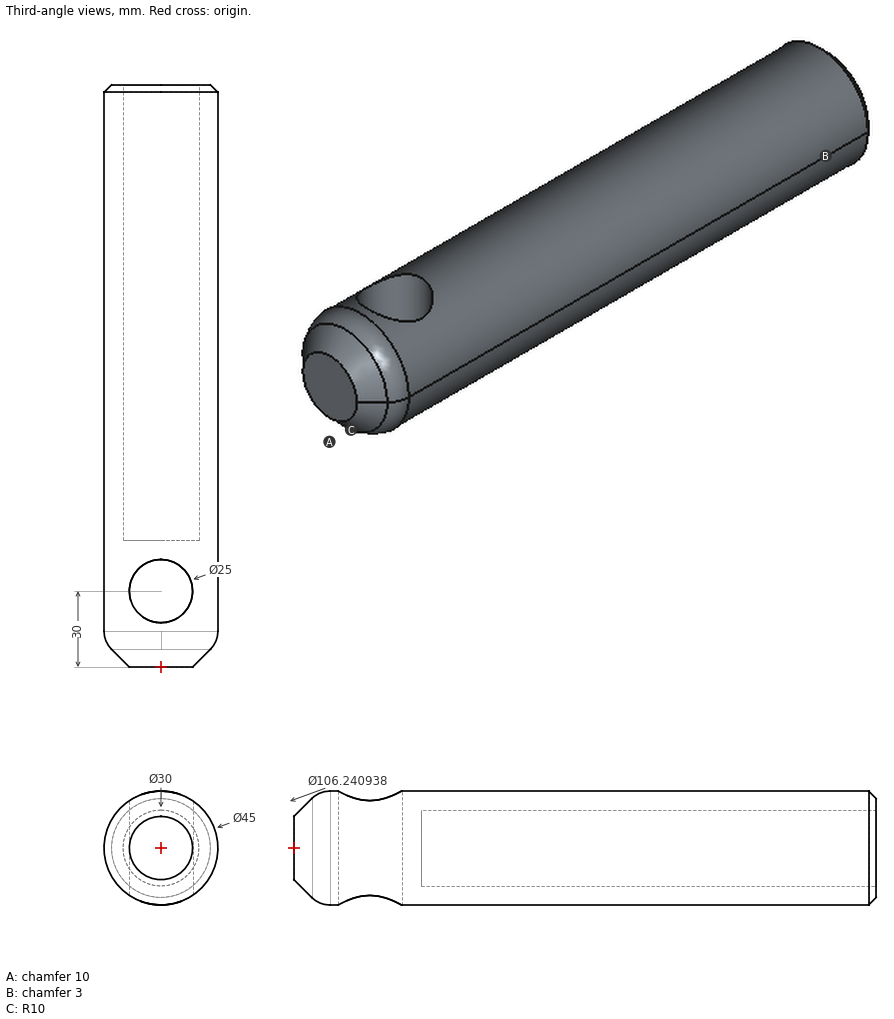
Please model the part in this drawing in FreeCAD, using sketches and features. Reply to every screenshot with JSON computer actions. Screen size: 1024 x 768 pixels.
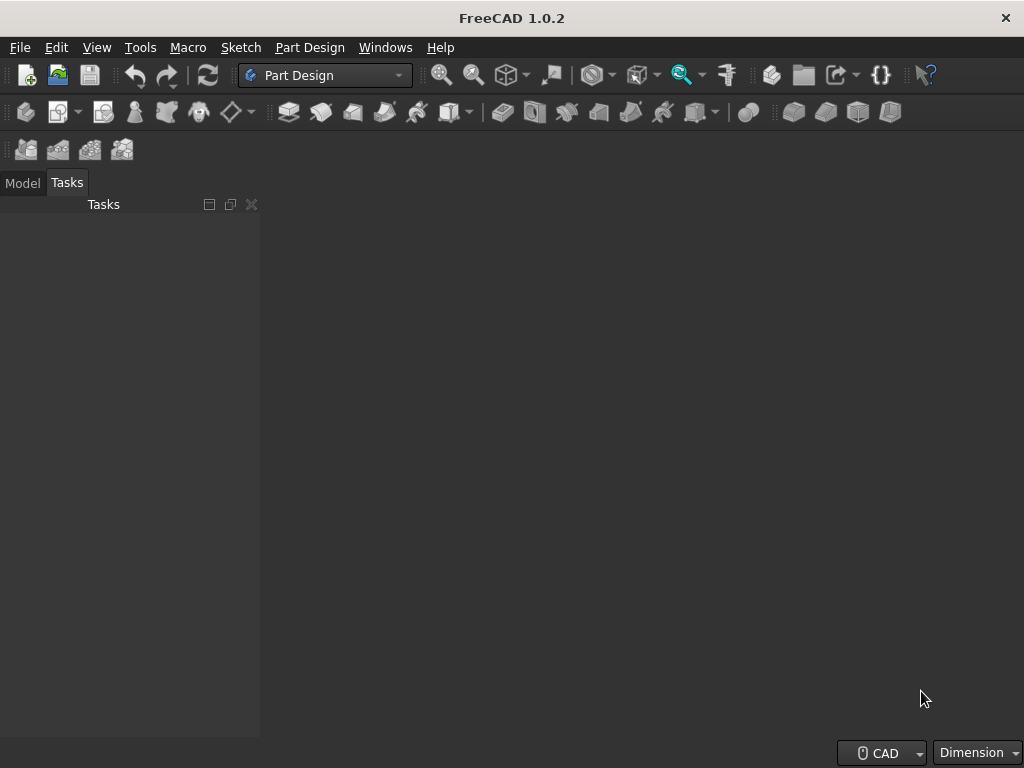
{"action": "key", "text": "ctrl+n"}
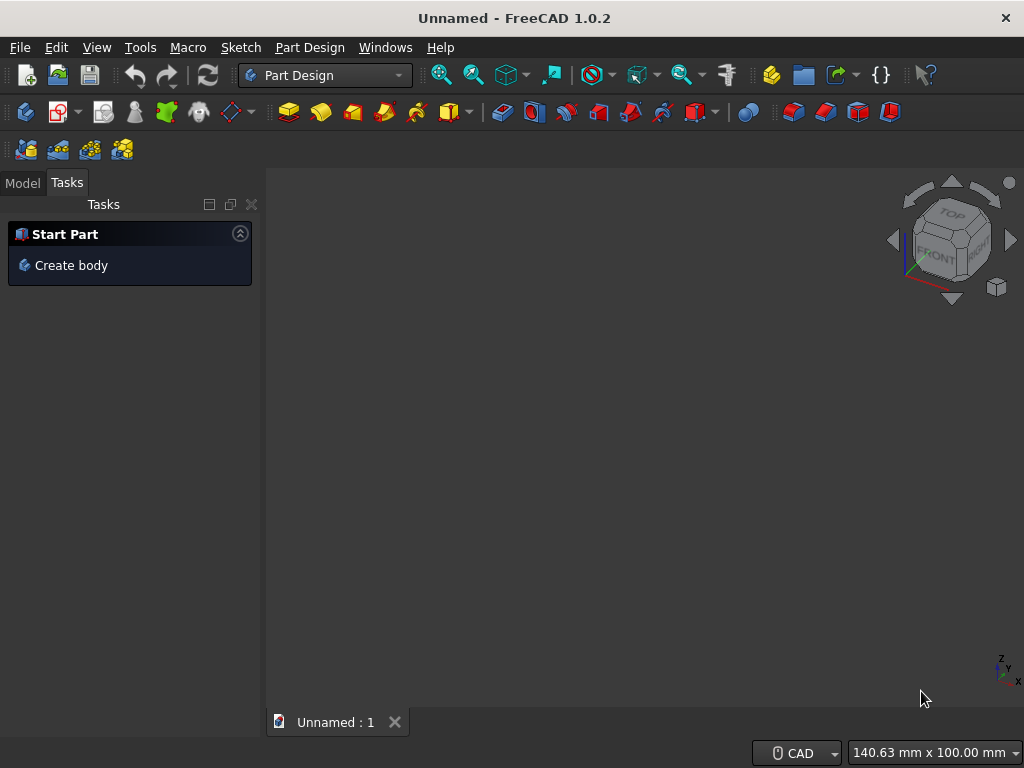
{"action": "left_click", "coordinate": [58, 112]}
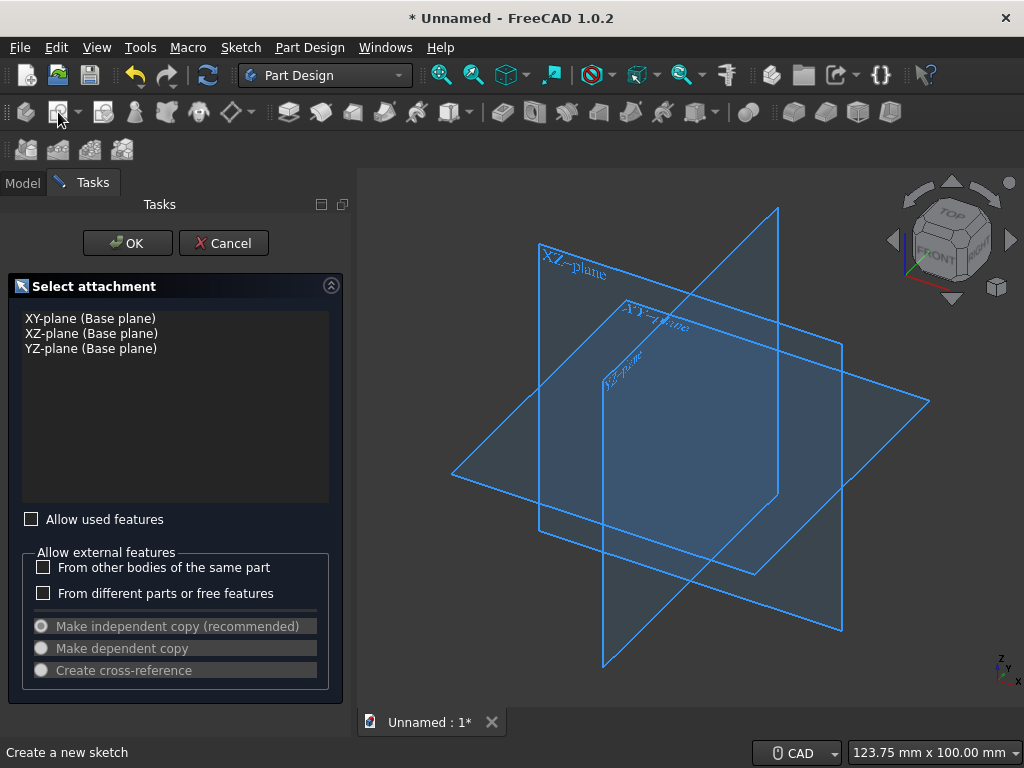
{"action": "left_click", "coordinate": [82, 334]}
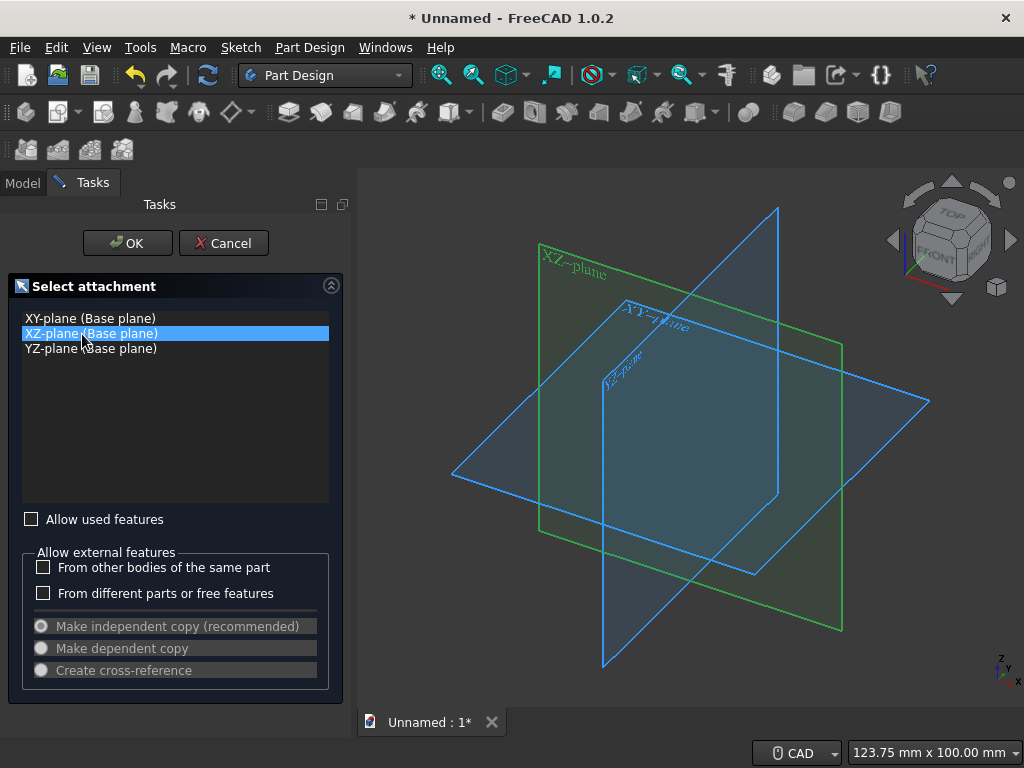
{"action": "left_click", "coordinate": [128, 243]}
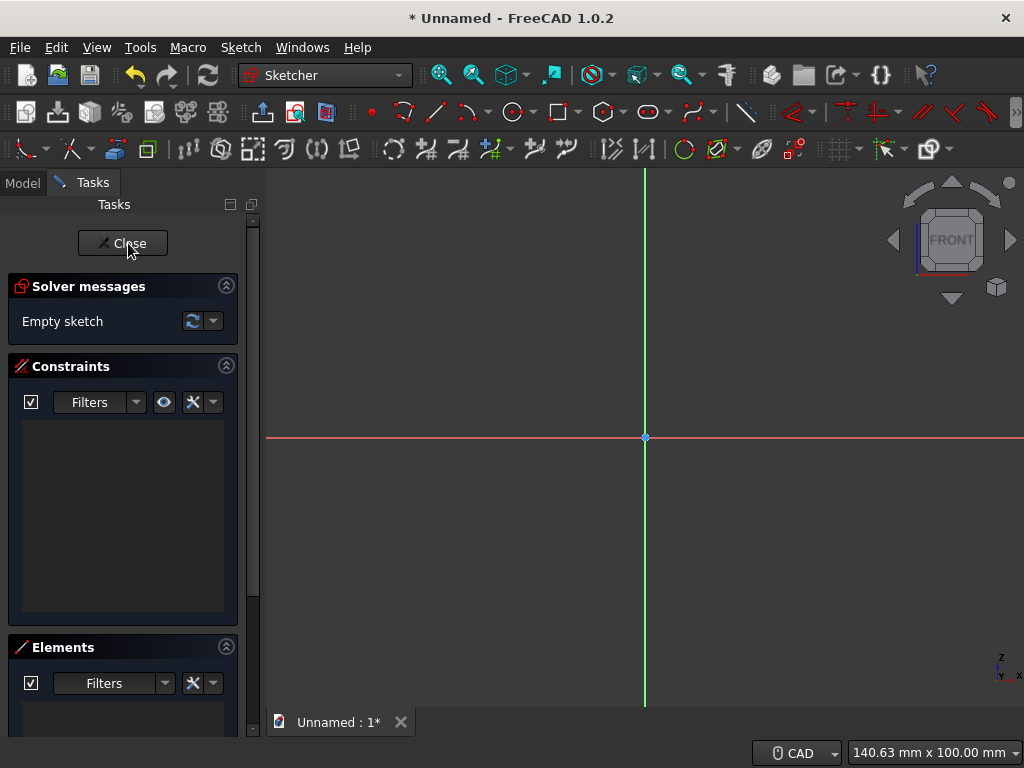
{"action": "scroll", "coordinate": [784, 438], "scroll_direction": "up", "scroll_amount": 2}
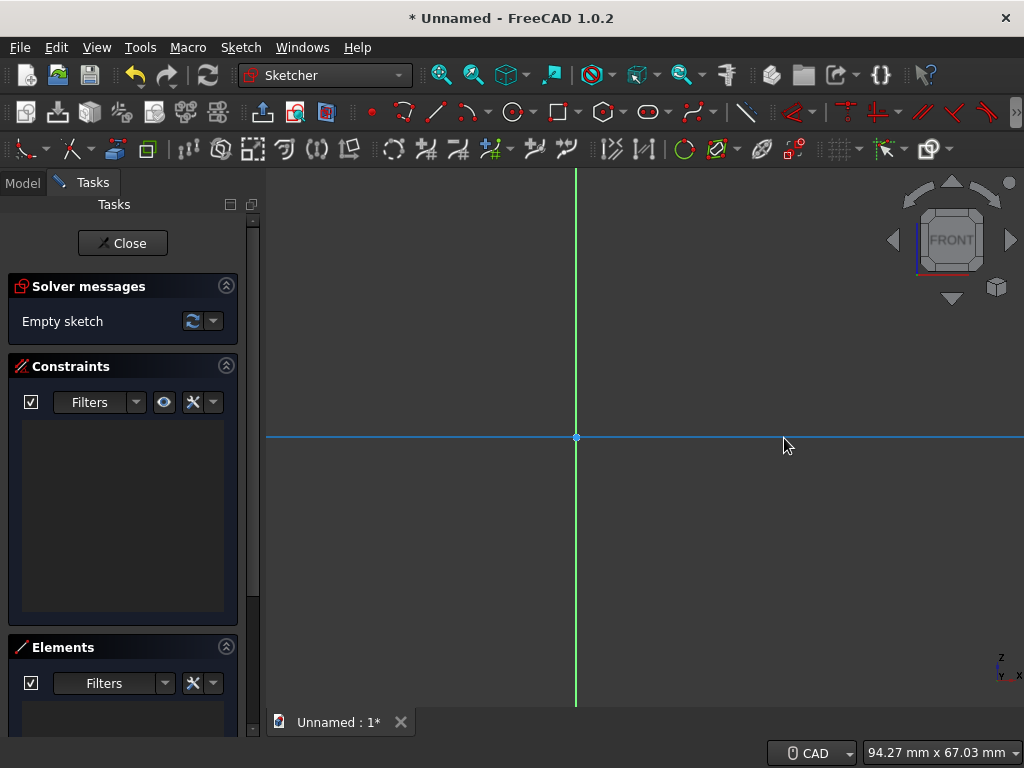
{"action": "left_click", "coordinate": [514, 112]}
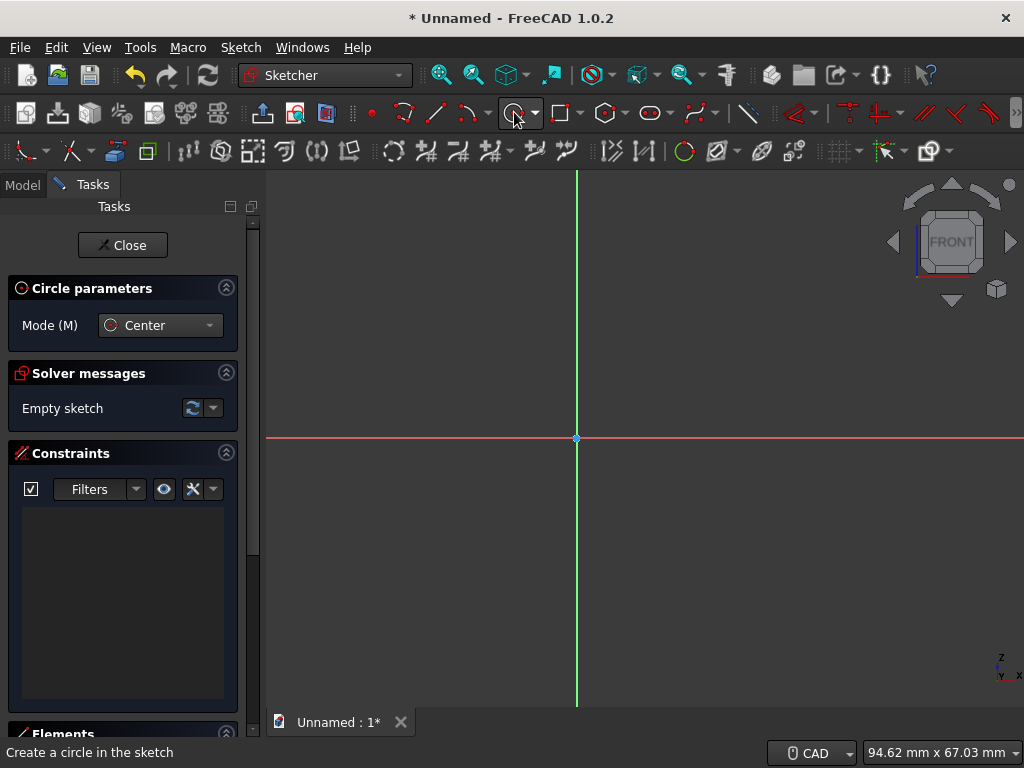
{"action": "left_click", "coordinate": [577, 438]}
{"action": "mouse_move", "coordinate": [704, 311]}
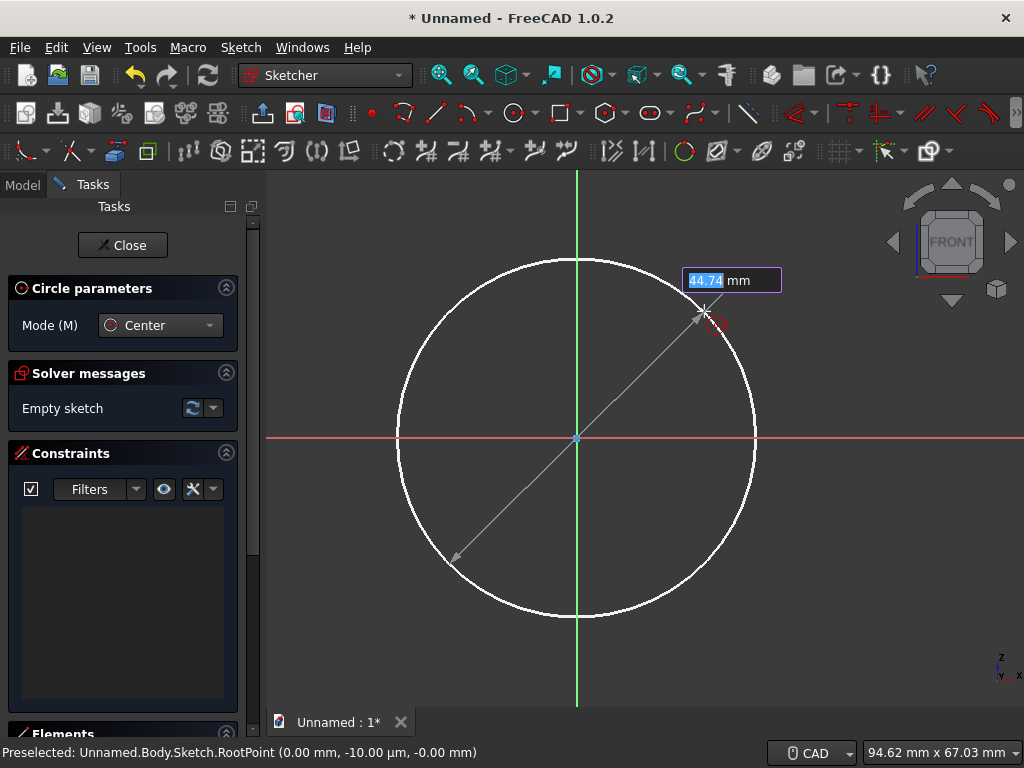
{"action": "type", "text": "45"}
{"action": "key", "text": "Return"}
{"action": "key", "text": "Escape"}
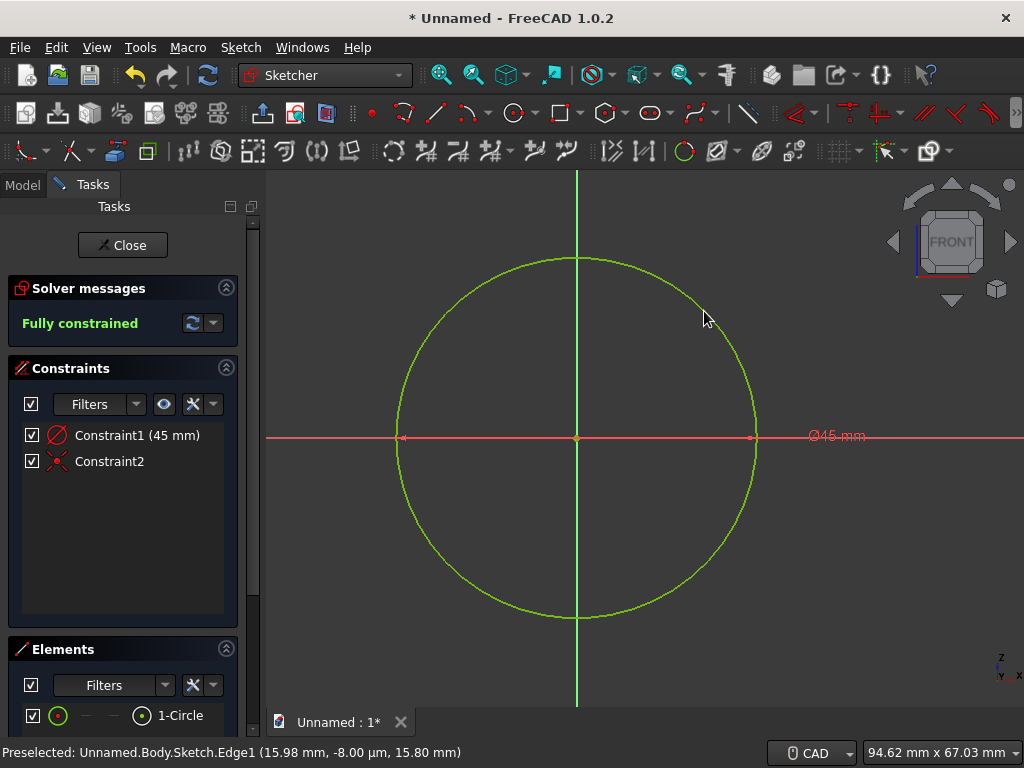
{"action": "left_click", "coordinate": [123, 245]}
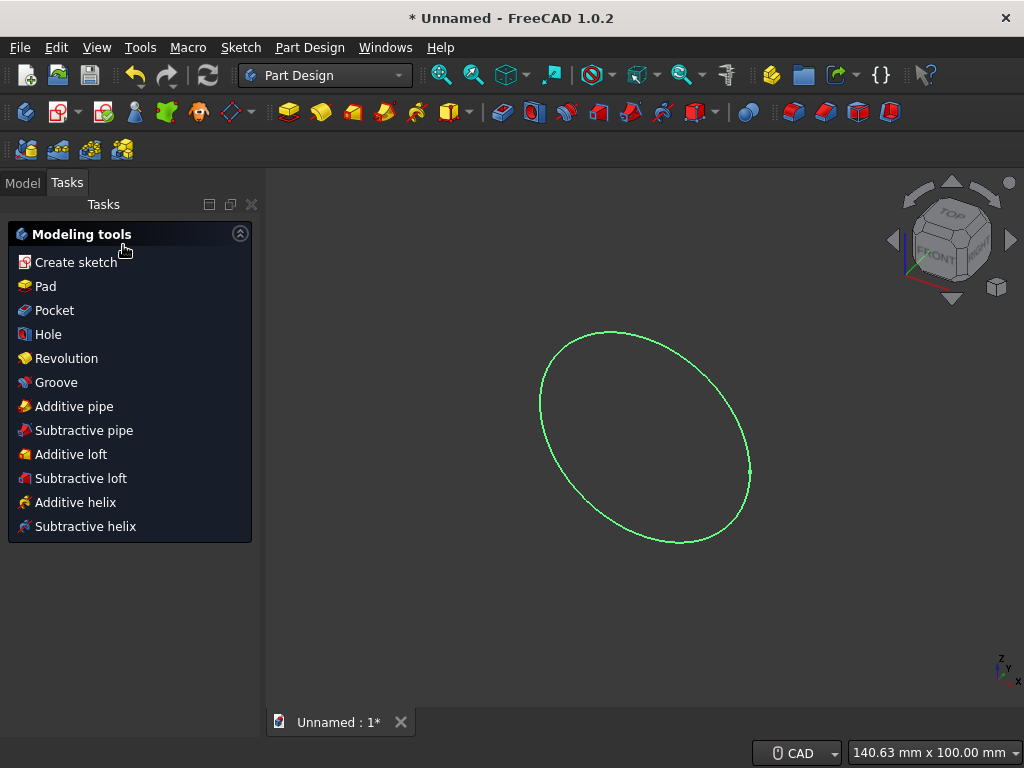
{"action": "left_click", "coordinate": [290, 112]}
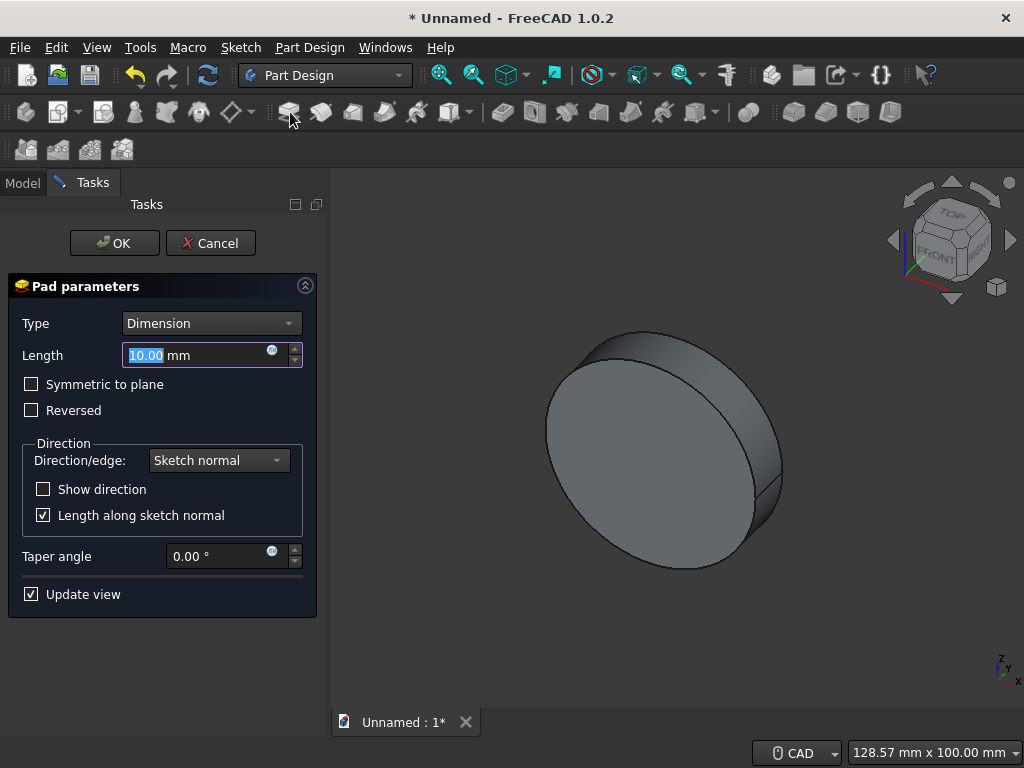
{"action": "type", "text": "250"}
{"action": "key", "text": "Tab"}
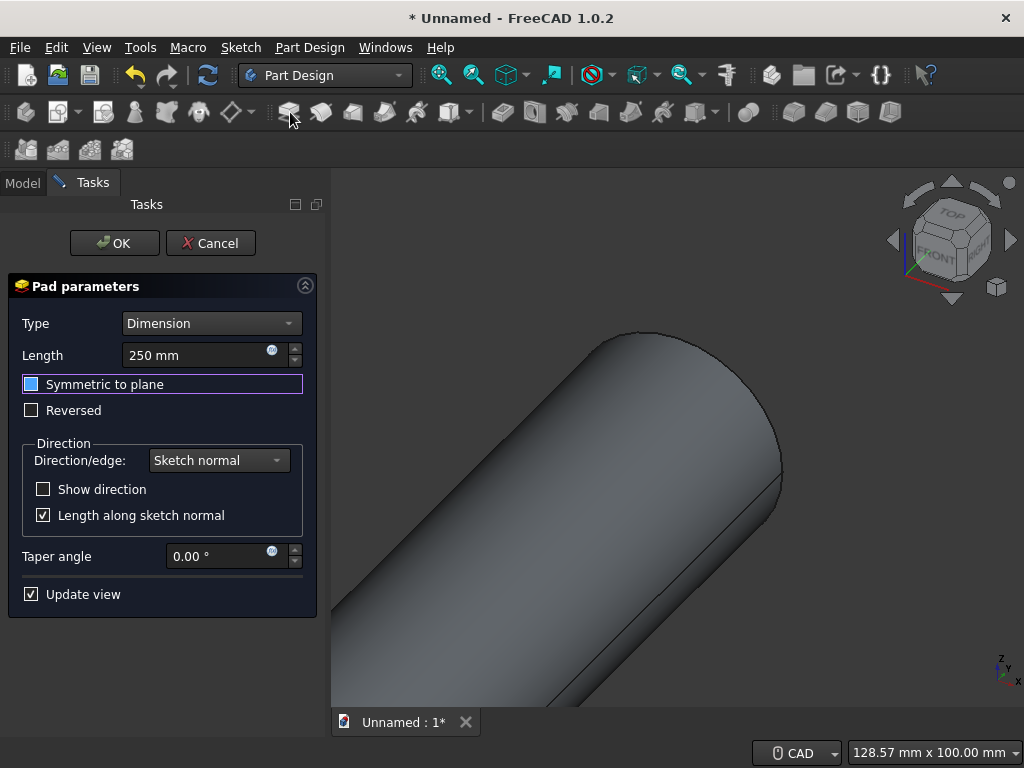
{"action": "left_click", "coordinate": [30, 410]}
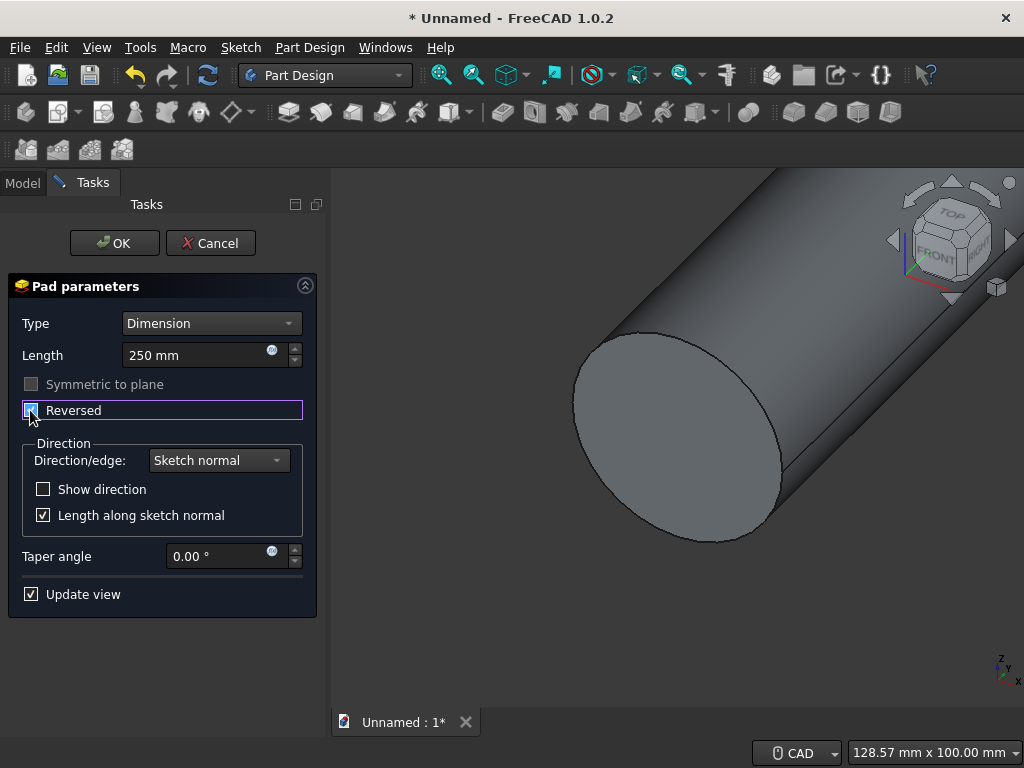
{"action": "left_click", "coordinate": [115, 243]}